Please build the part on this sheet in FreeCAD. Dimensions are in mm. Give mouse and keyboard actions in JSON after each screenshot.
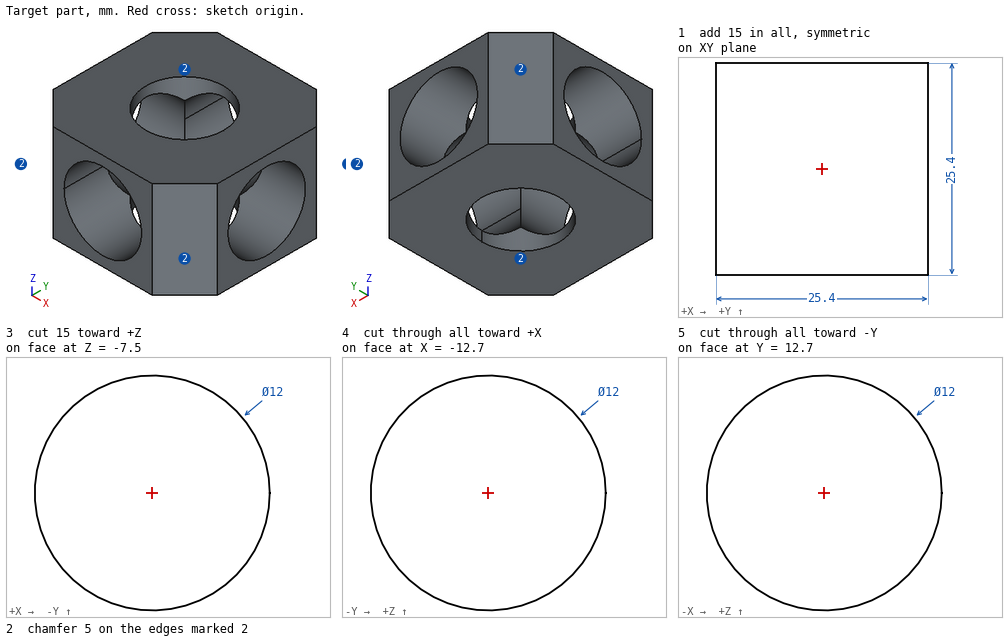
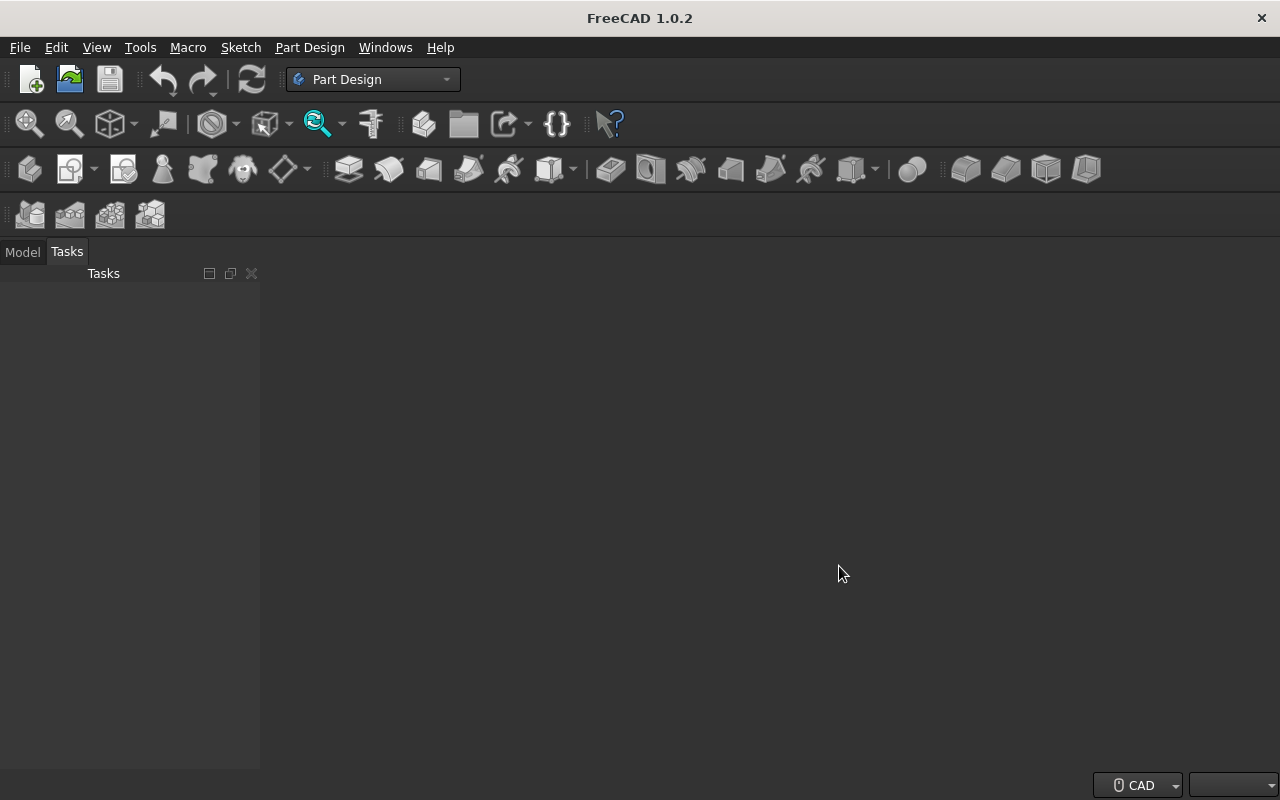
{"action": "key", "text": "ctrl+n"}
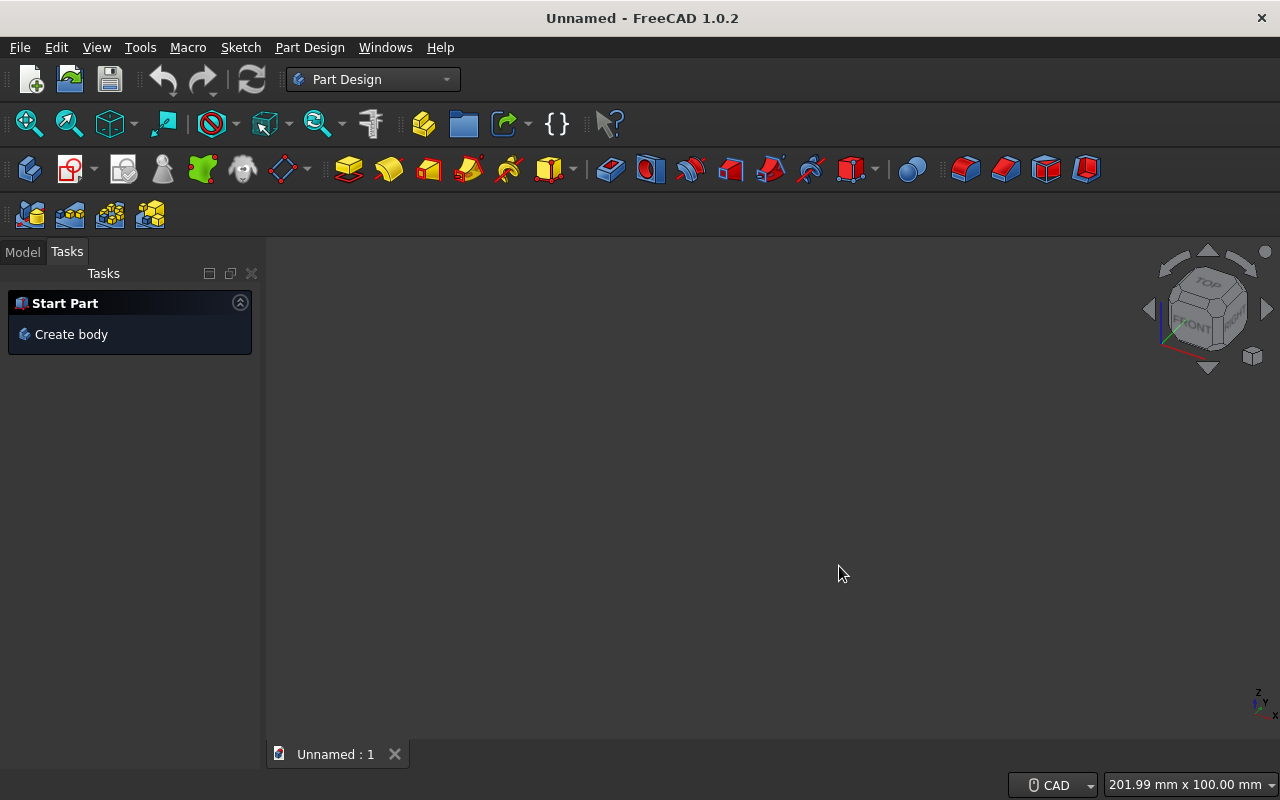
{"action": "left_click", "coordinate": [70, 170]}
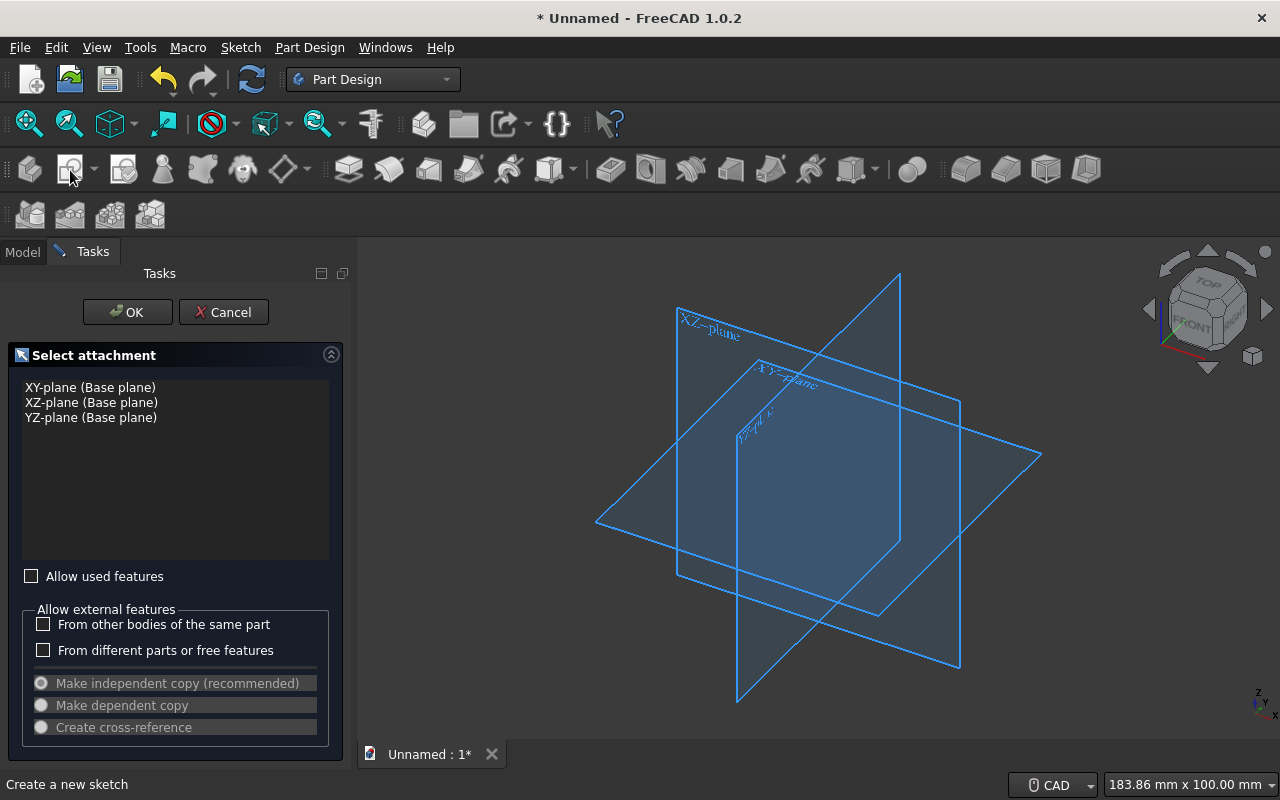
{"action": "left_click", "coordinate": [82, 388]}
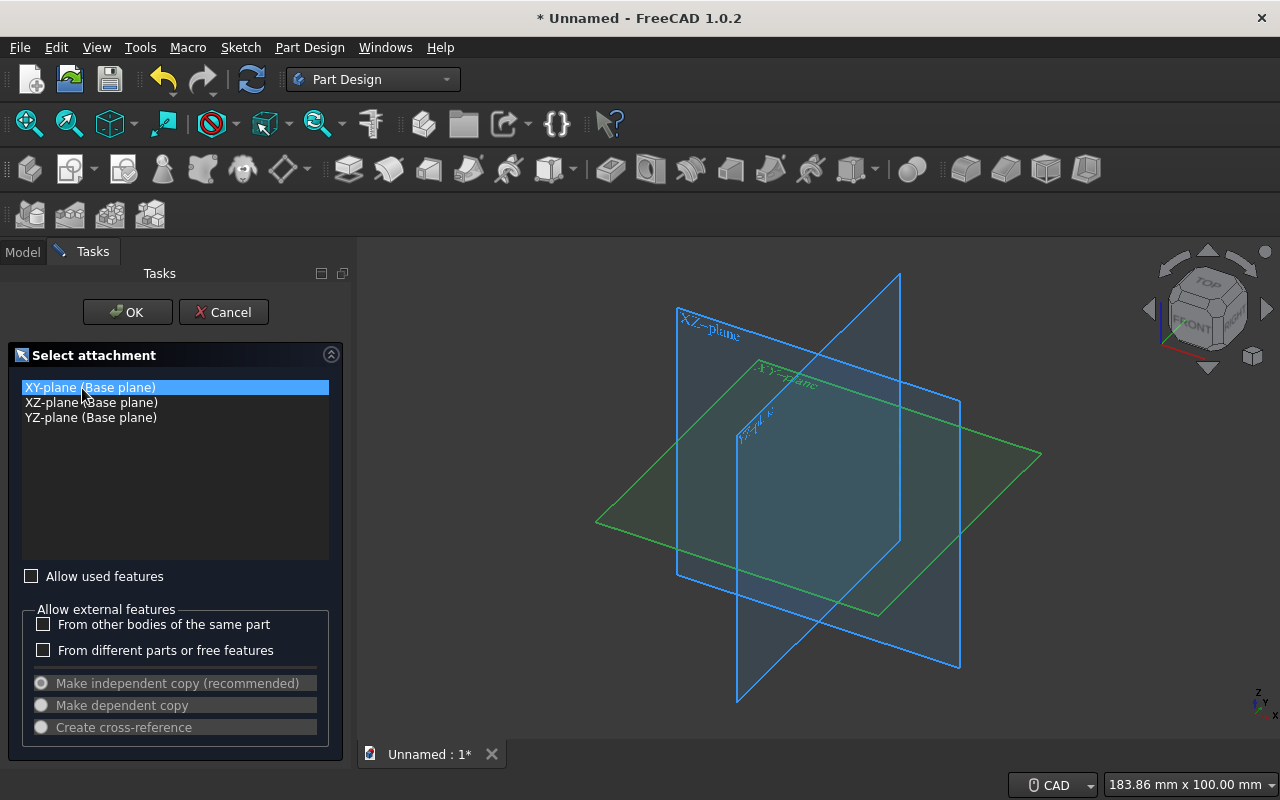
{"action": "left_click", "coordinate": [128, 312]}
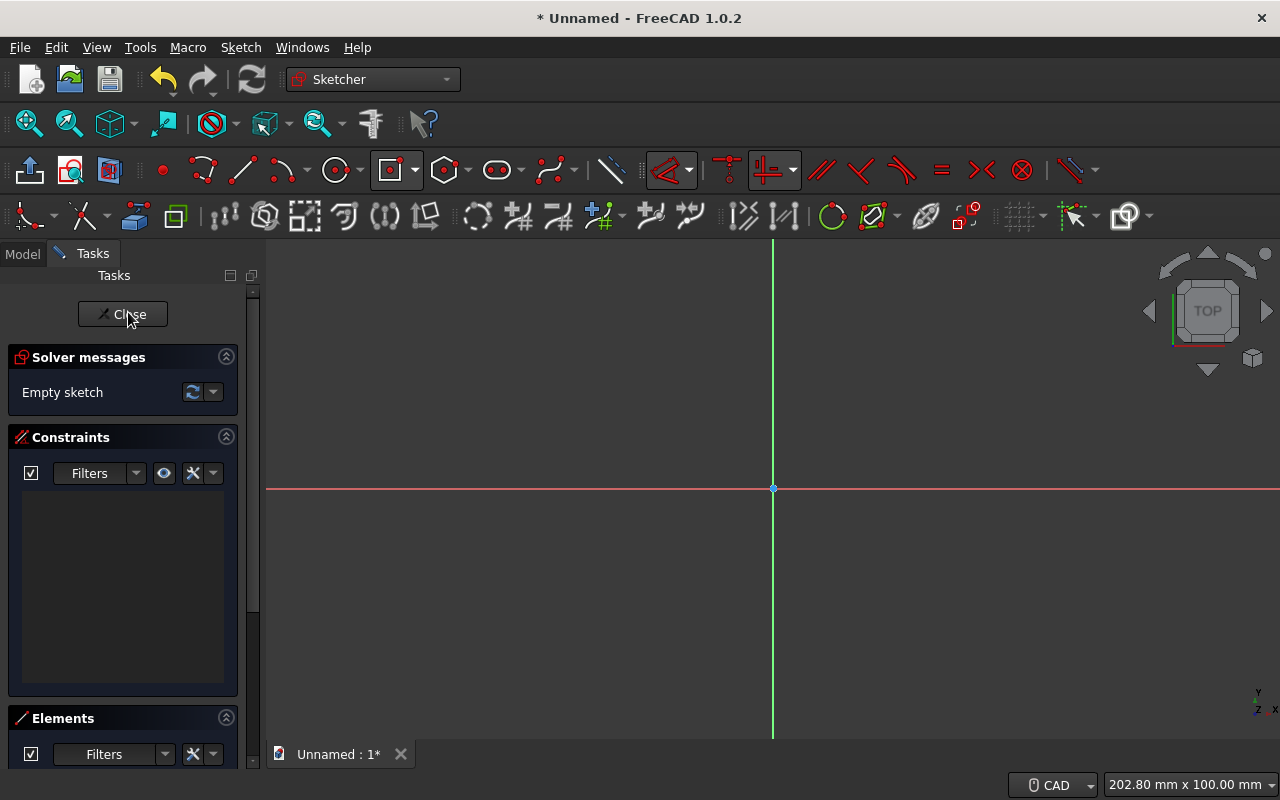
{"action": "scroll", "coordinate": [813, 489], "scroll_direction": "up", "scroll_amount": 5}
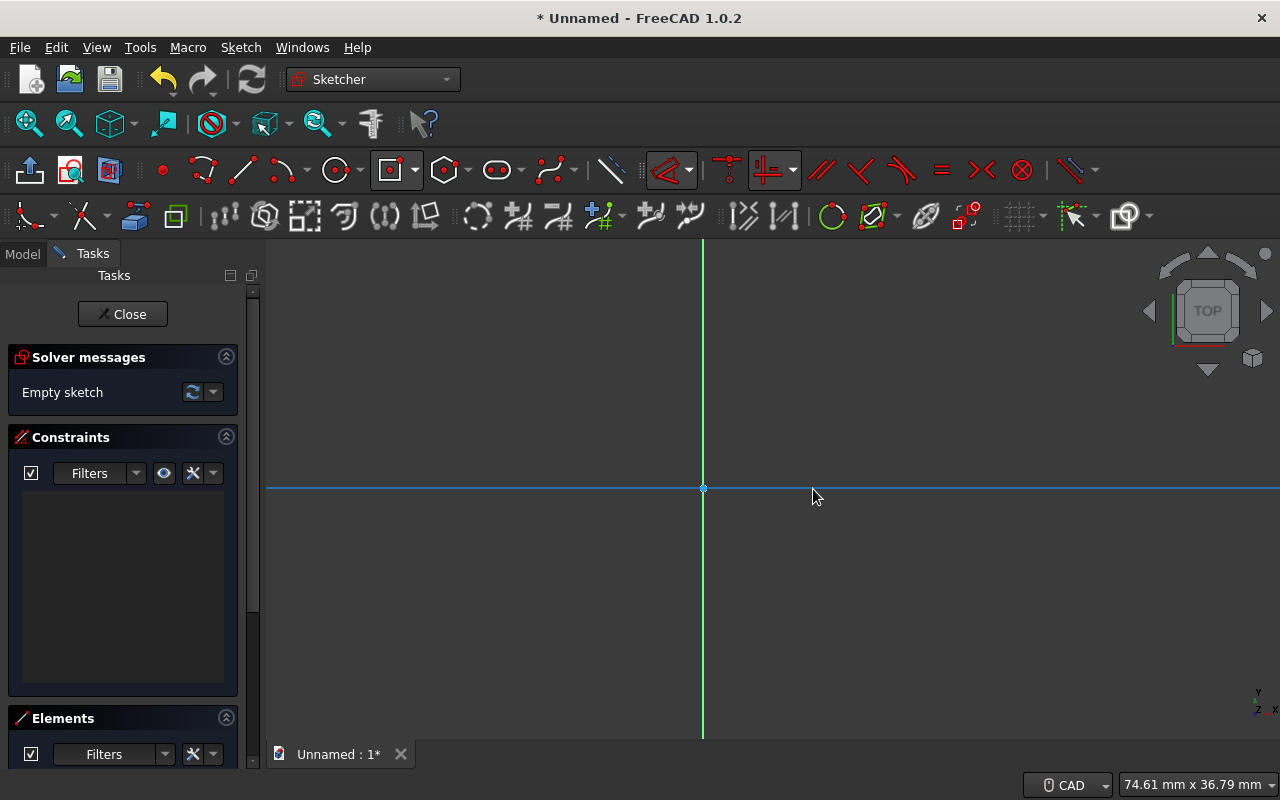
{"action": "left_click", "coordinate": [390, 170]}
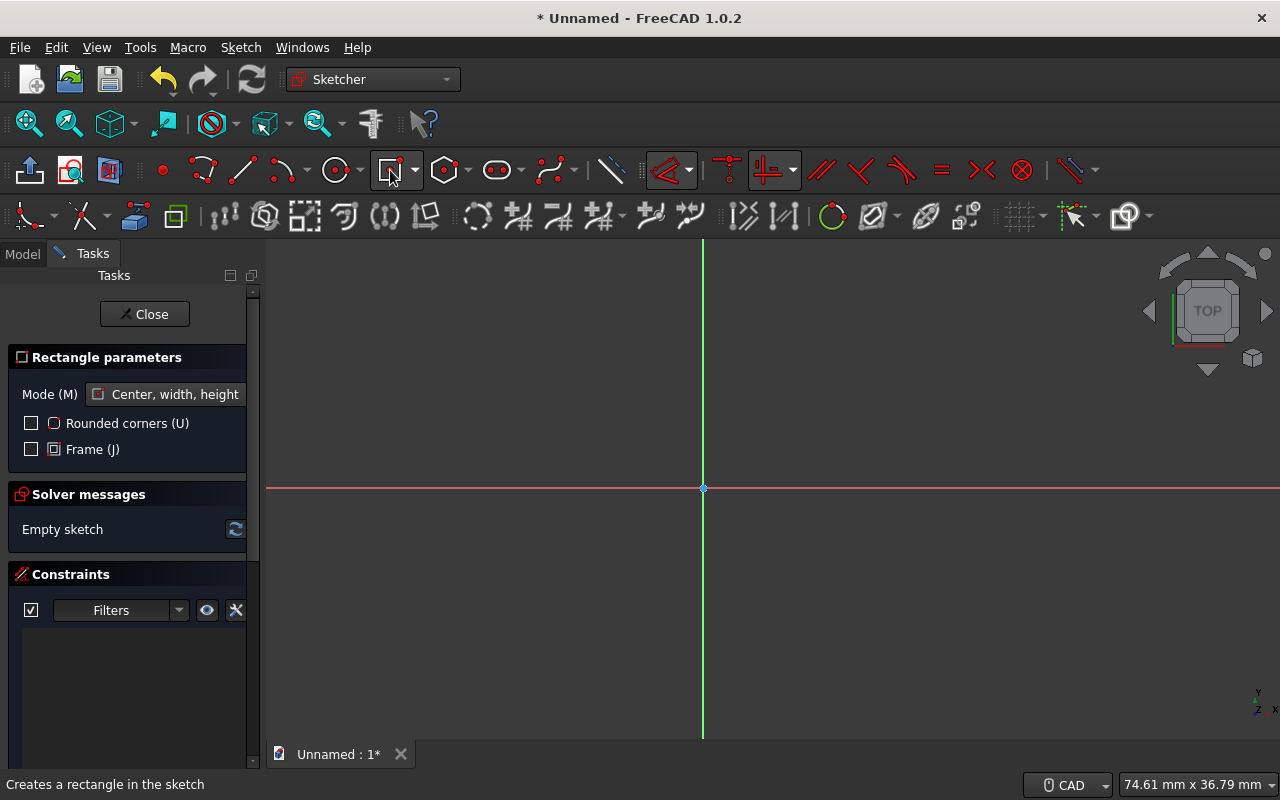
{"action": "left_click", "coordinate": [703, 488]}
{"action": "left_click", "coordinate": [876, 316]}
{"action": "key", "text": "Escape"}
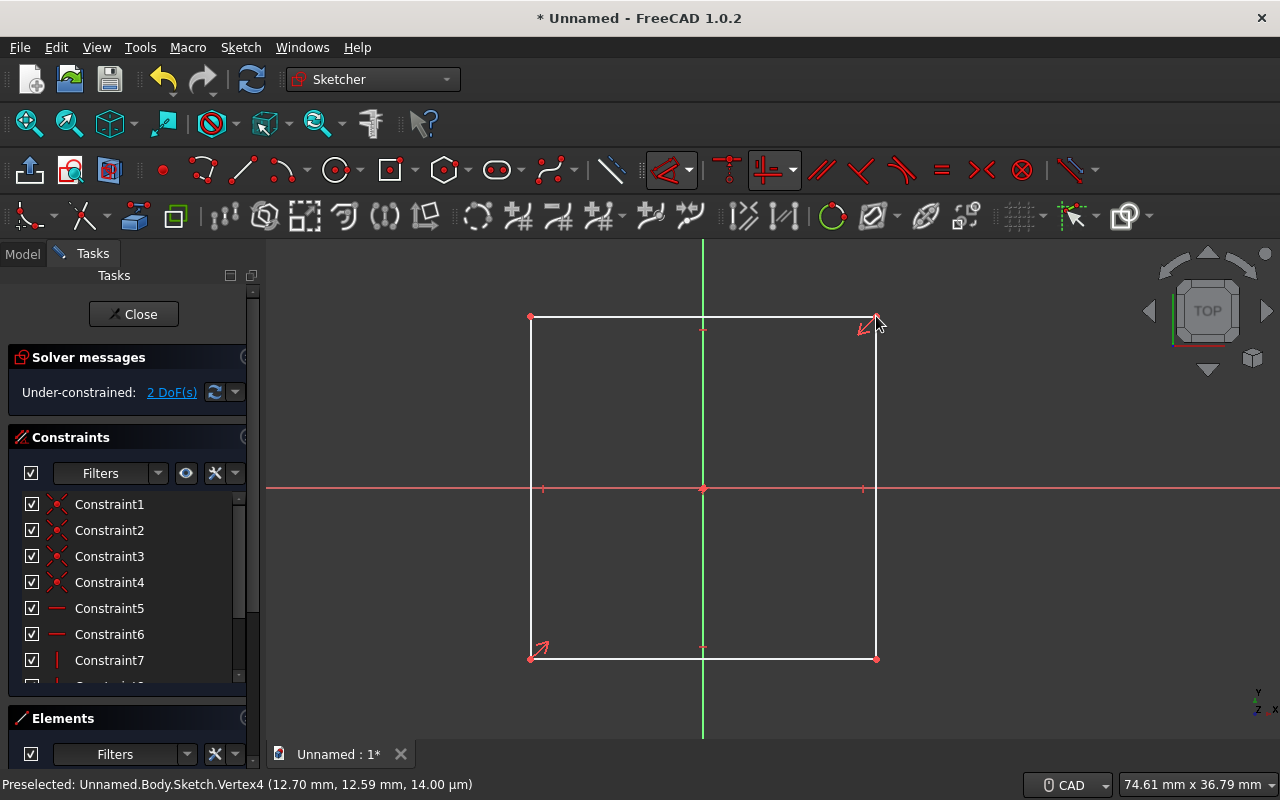
{"action": "key", "text": "d"}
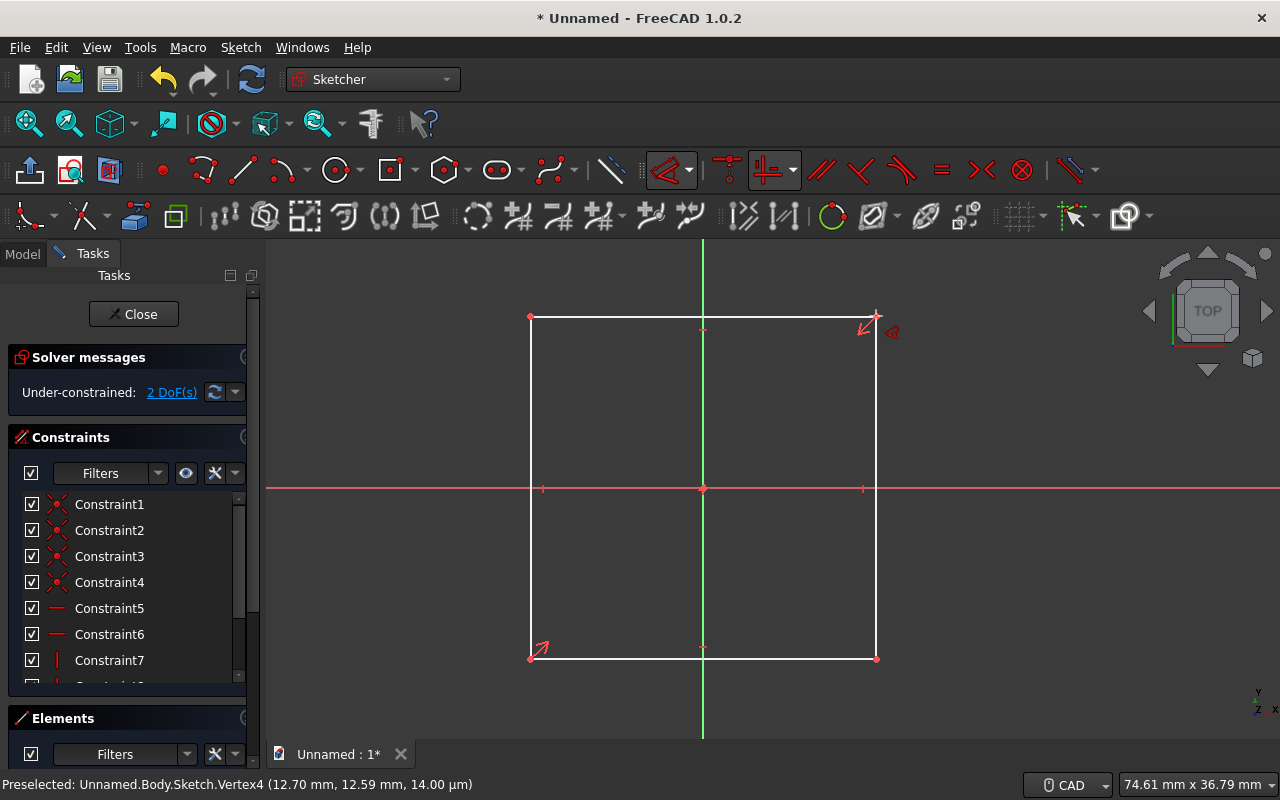
{"action": "left_click", "coordinate": [634, 659]}
{"action": "left_click", "coordinate": [624, 693]}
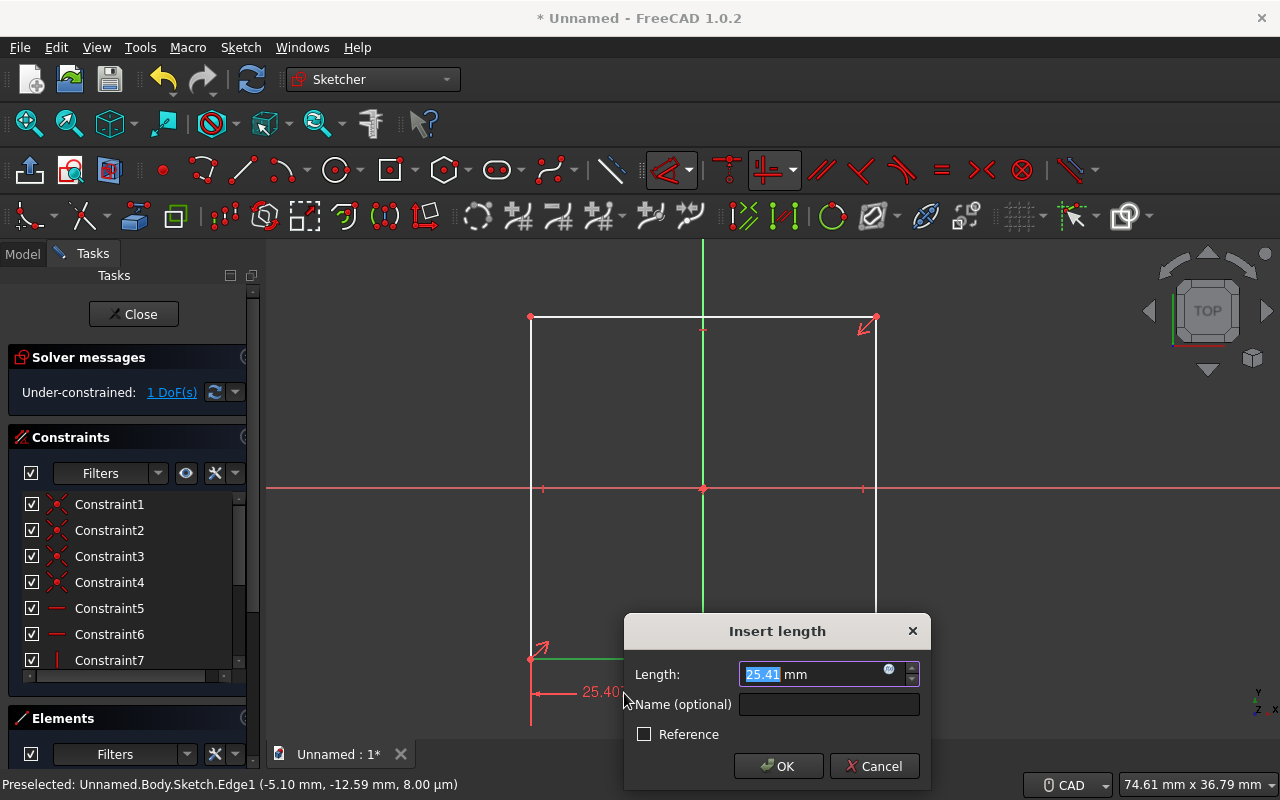
{"action": "type", "text": "25.4"}
{"action": "key", "text": "Return"}